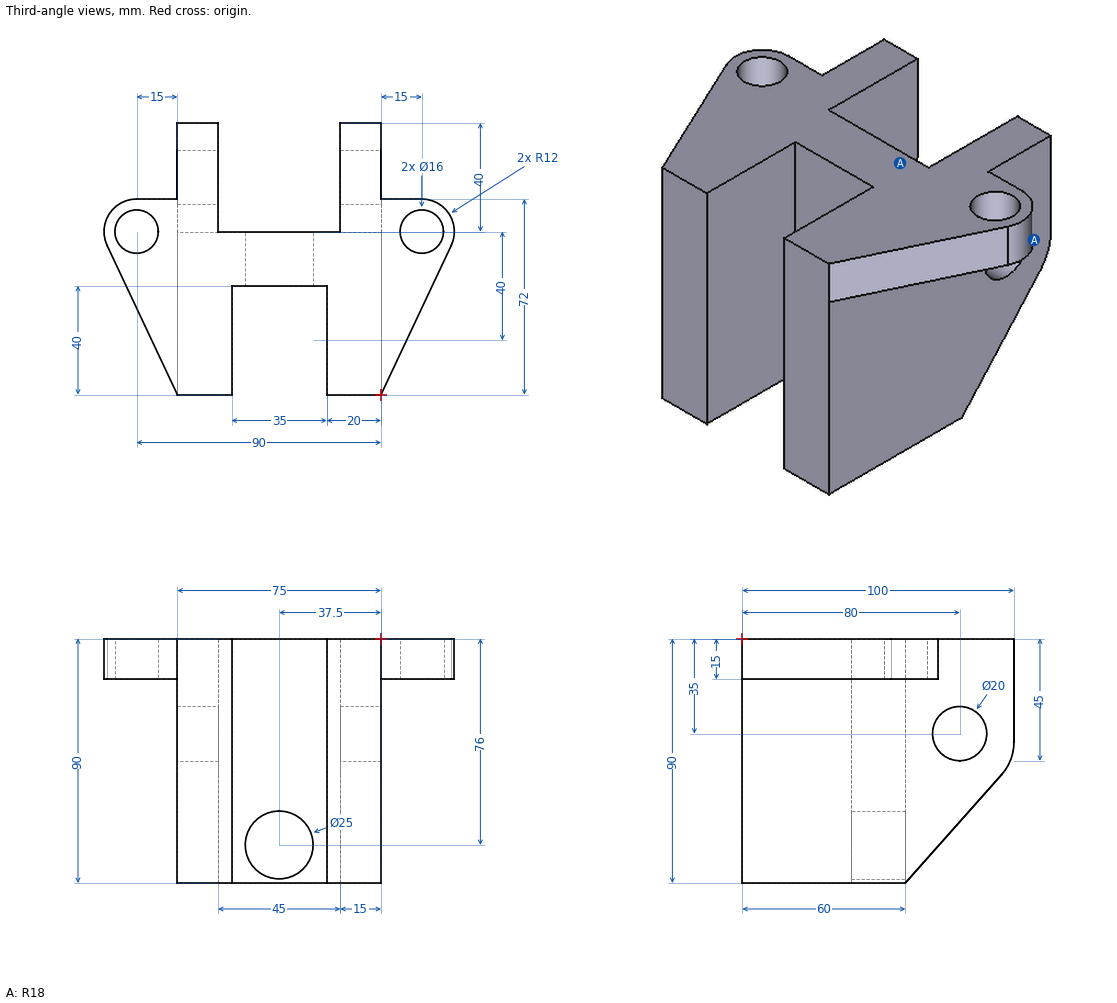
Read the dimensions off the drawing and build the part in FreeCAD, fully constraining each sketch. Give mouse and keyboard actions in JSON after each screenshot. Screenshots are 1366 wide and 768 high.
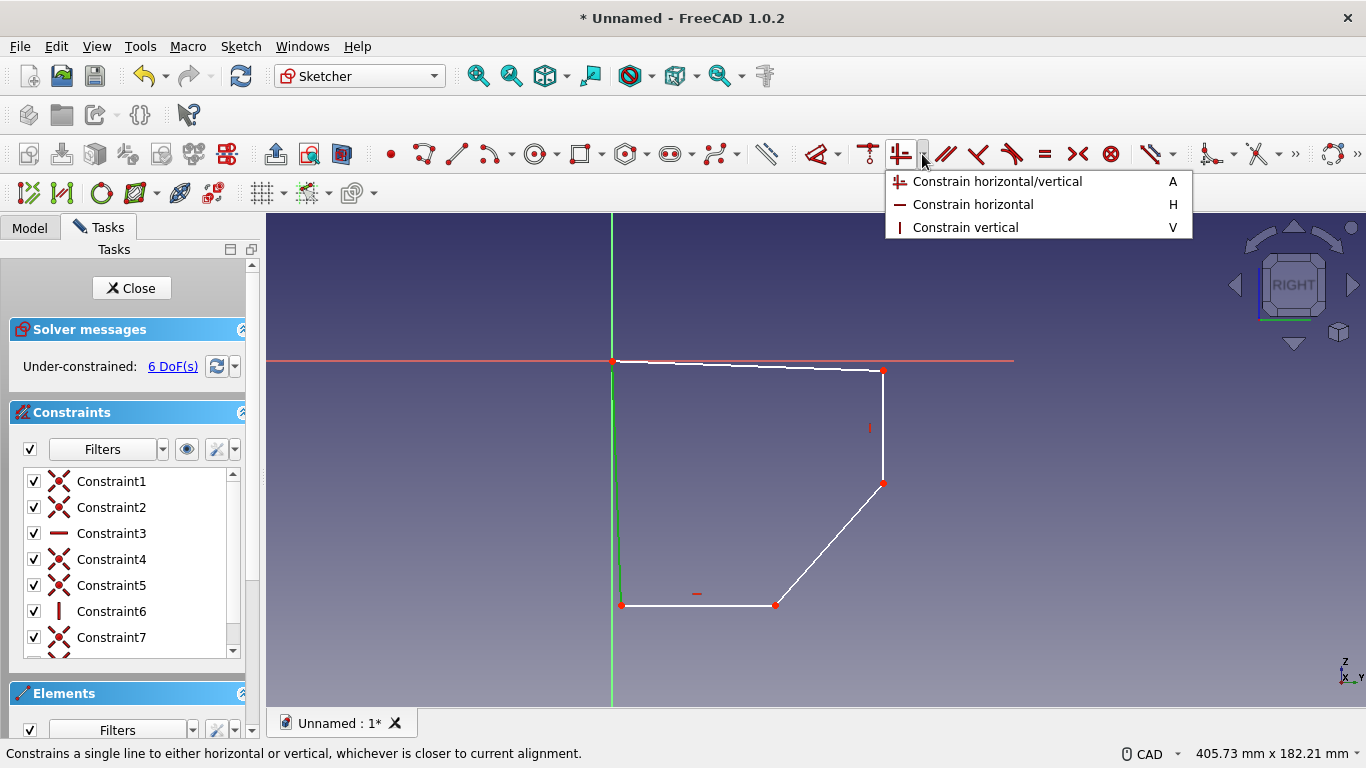
{"action": "left_click", "coordinate": [1039, 228]}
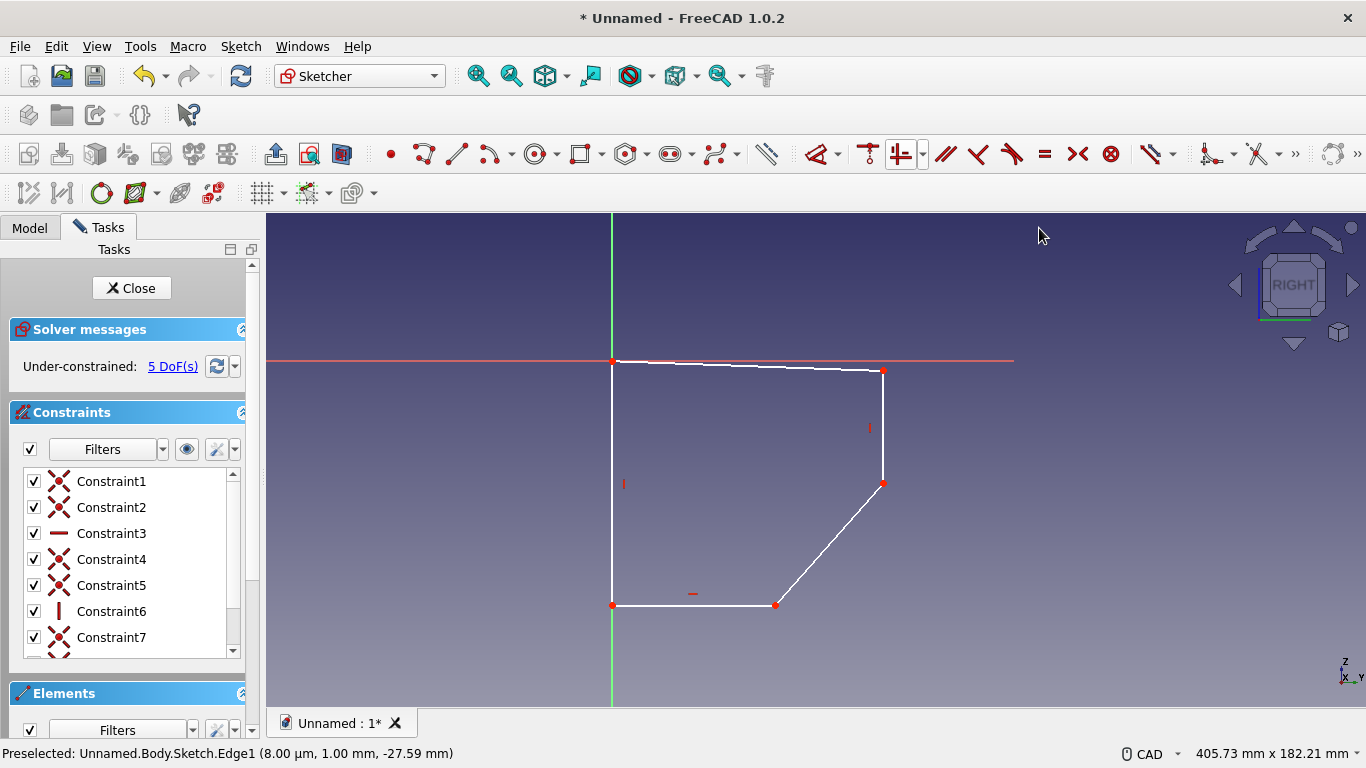
{"action": "left_click", "coordinate": [693, 364]}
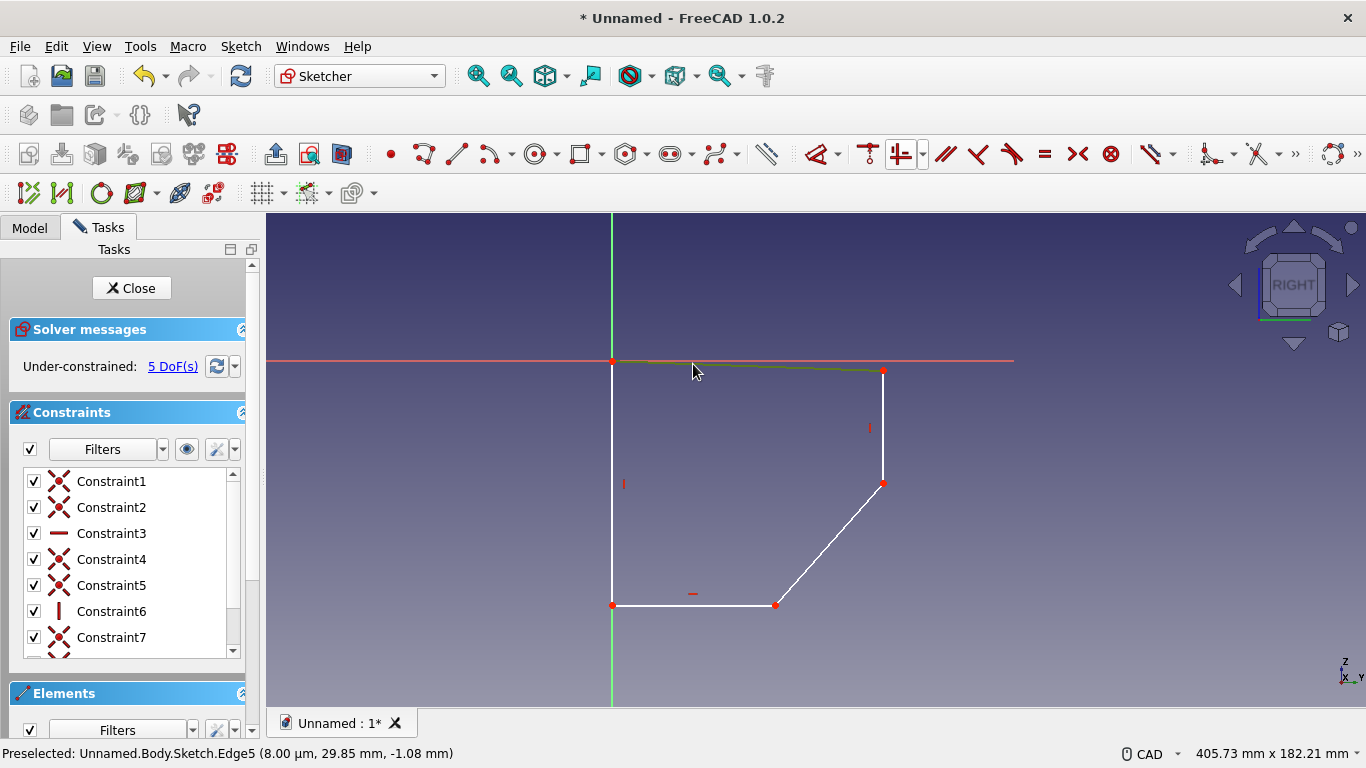
{"action": "key", "text": "h"}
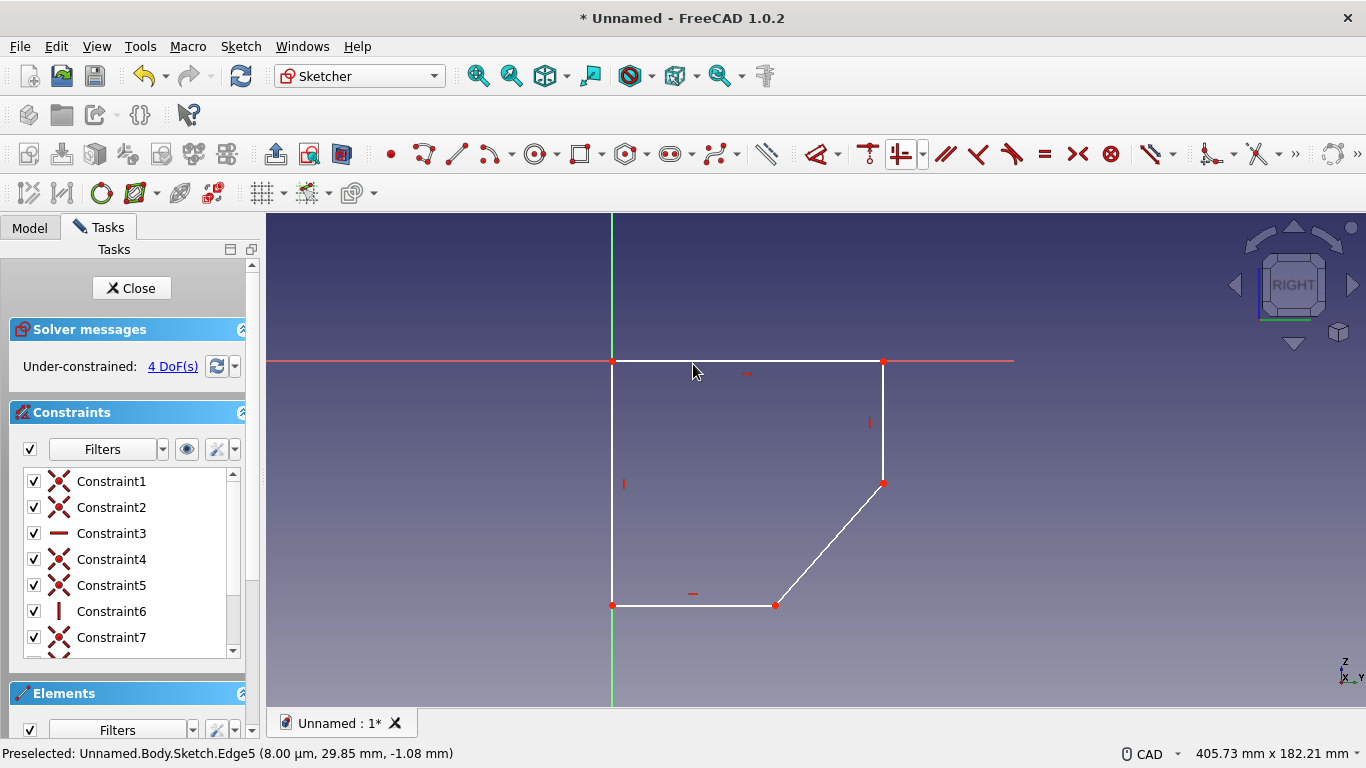
{"action": "left_click", "coordinate": [612, 435]}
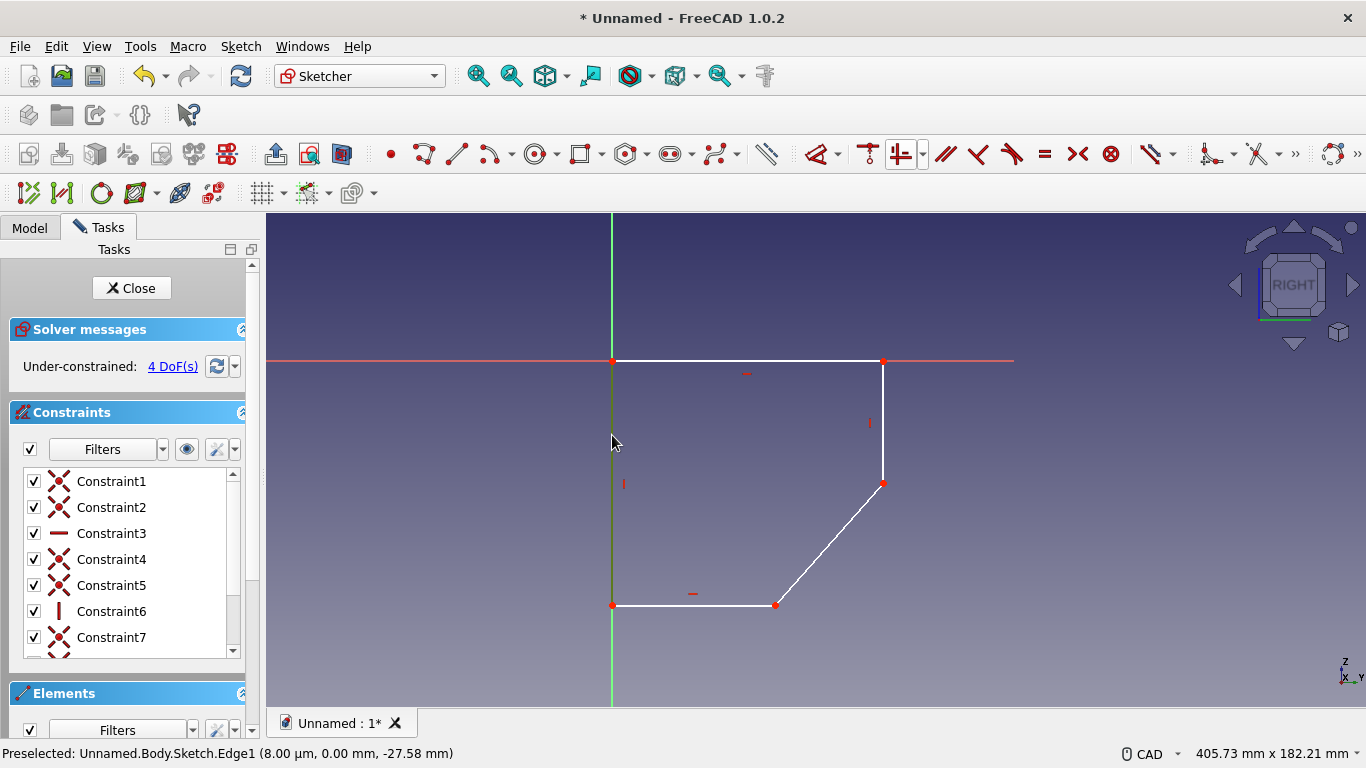
{"action": "key", "text": "i"}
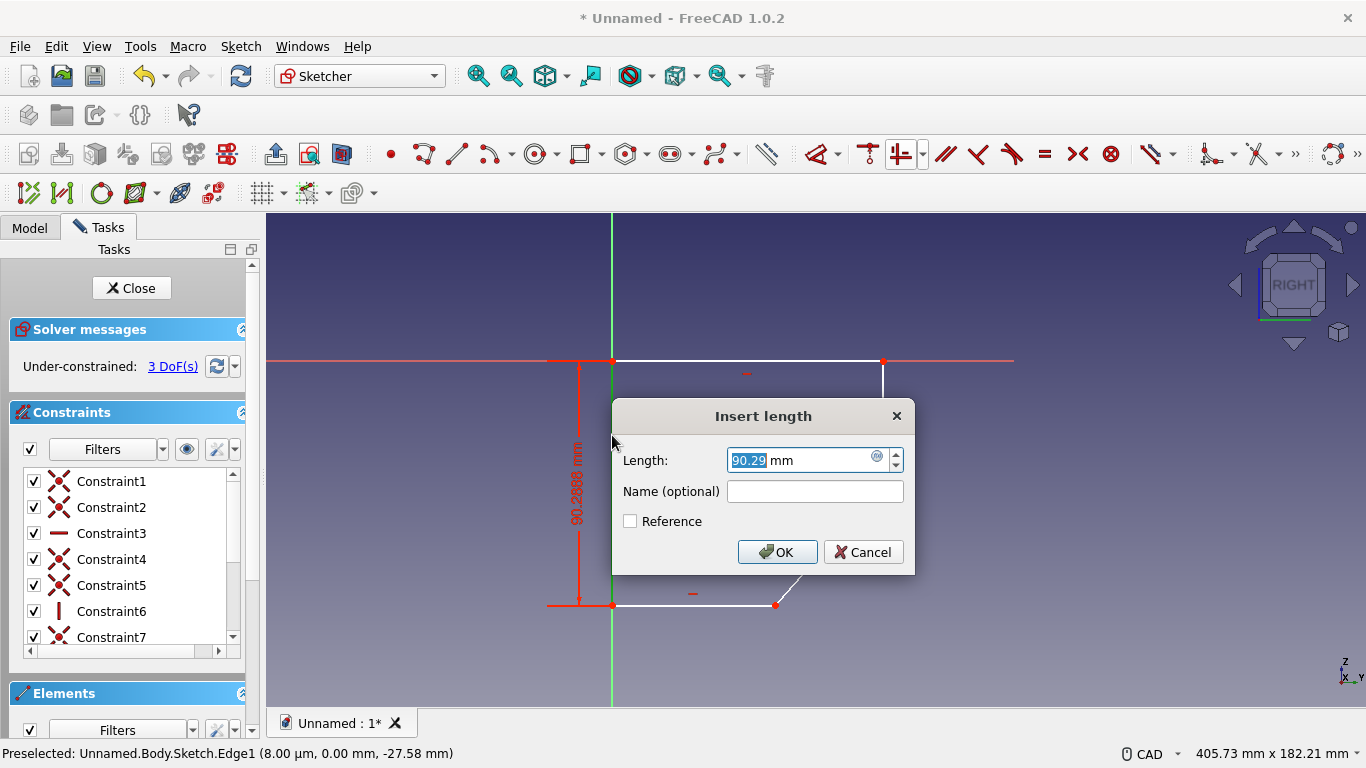
{"action": "type", "text": "90"}
{"action": "key", "text": "Return"}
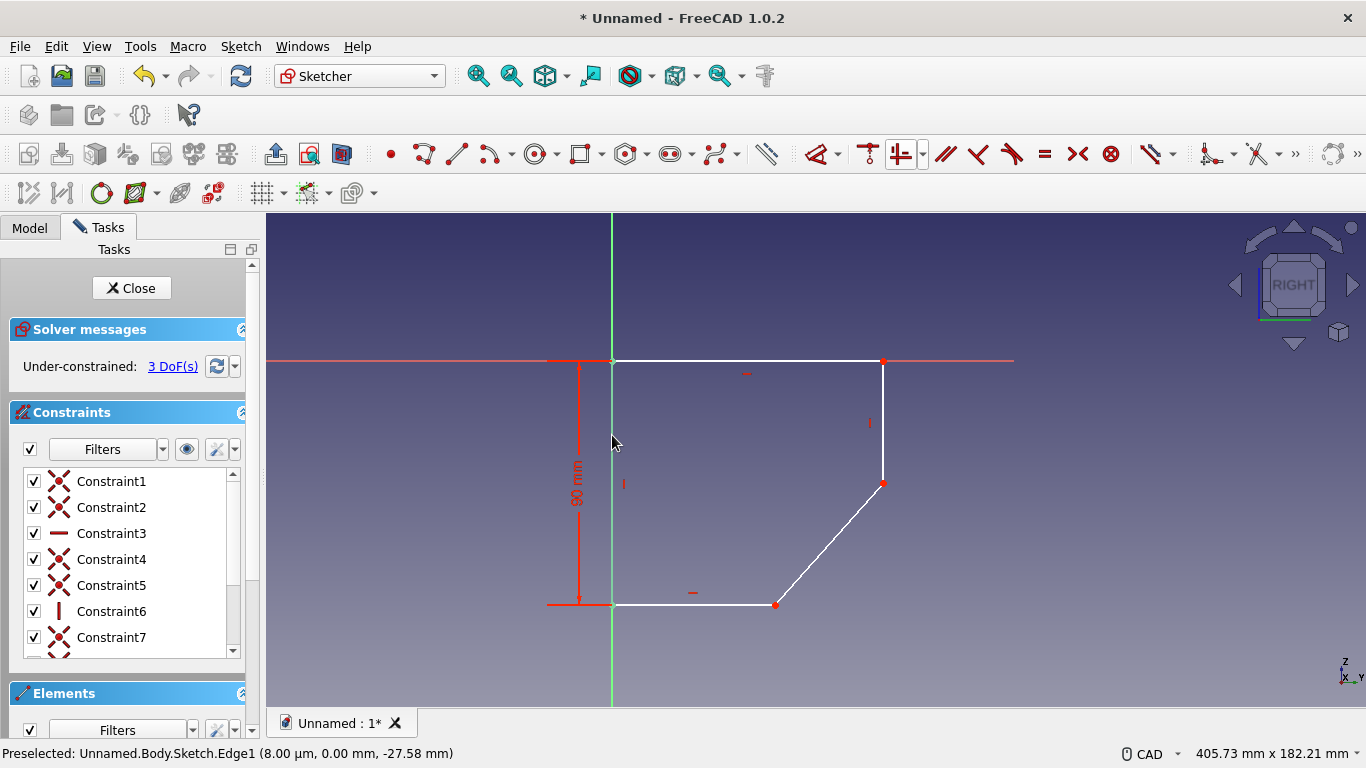
{"action": "left_click", "coordinate": [661, 605]}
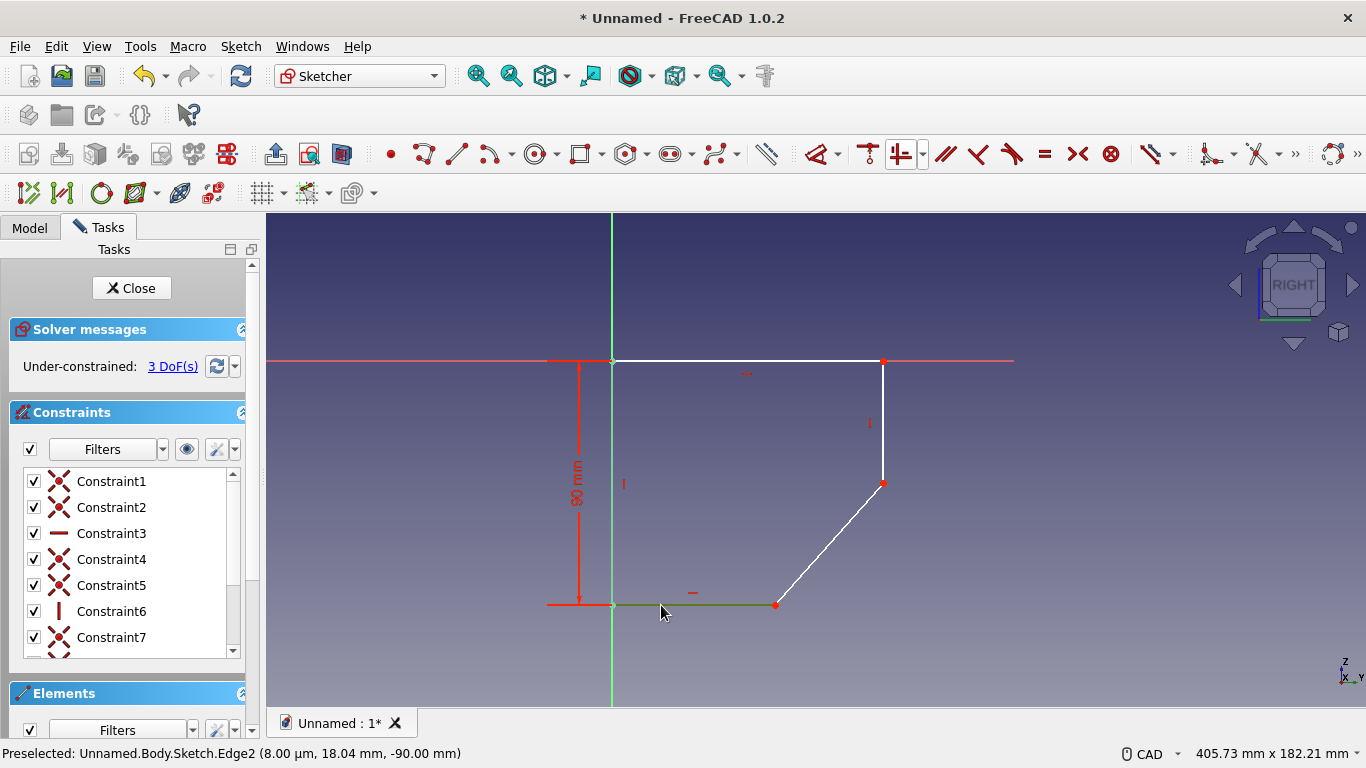
{"action": "left_click", "coordinate": [838, 154]}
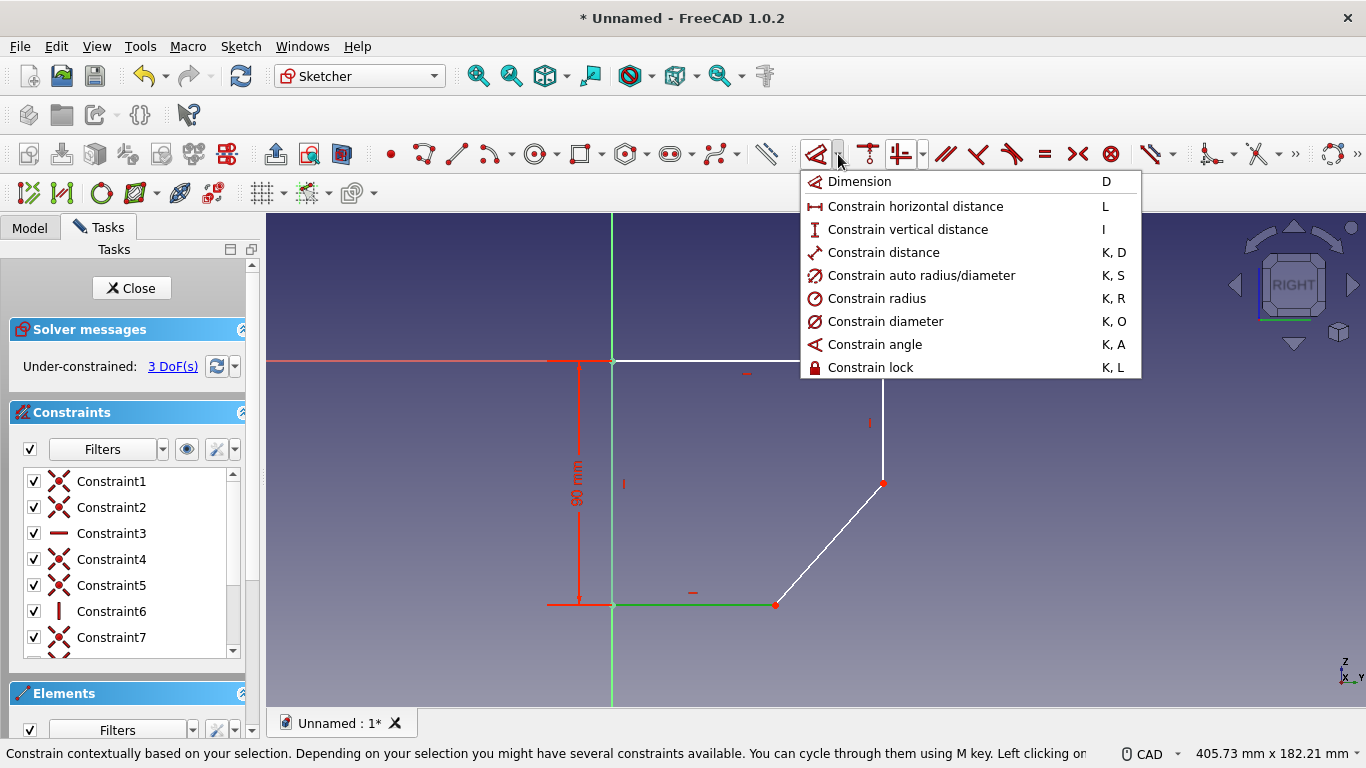
{"action": "left_click", "coordinate": [971, 206]}